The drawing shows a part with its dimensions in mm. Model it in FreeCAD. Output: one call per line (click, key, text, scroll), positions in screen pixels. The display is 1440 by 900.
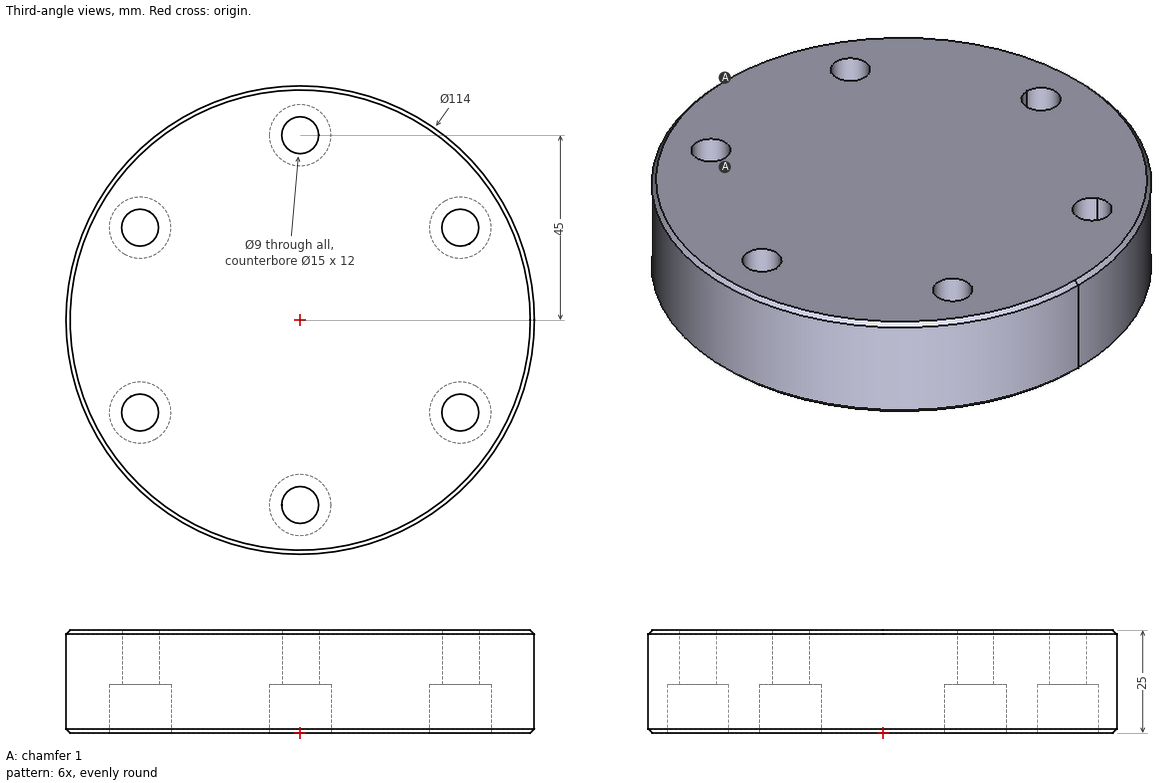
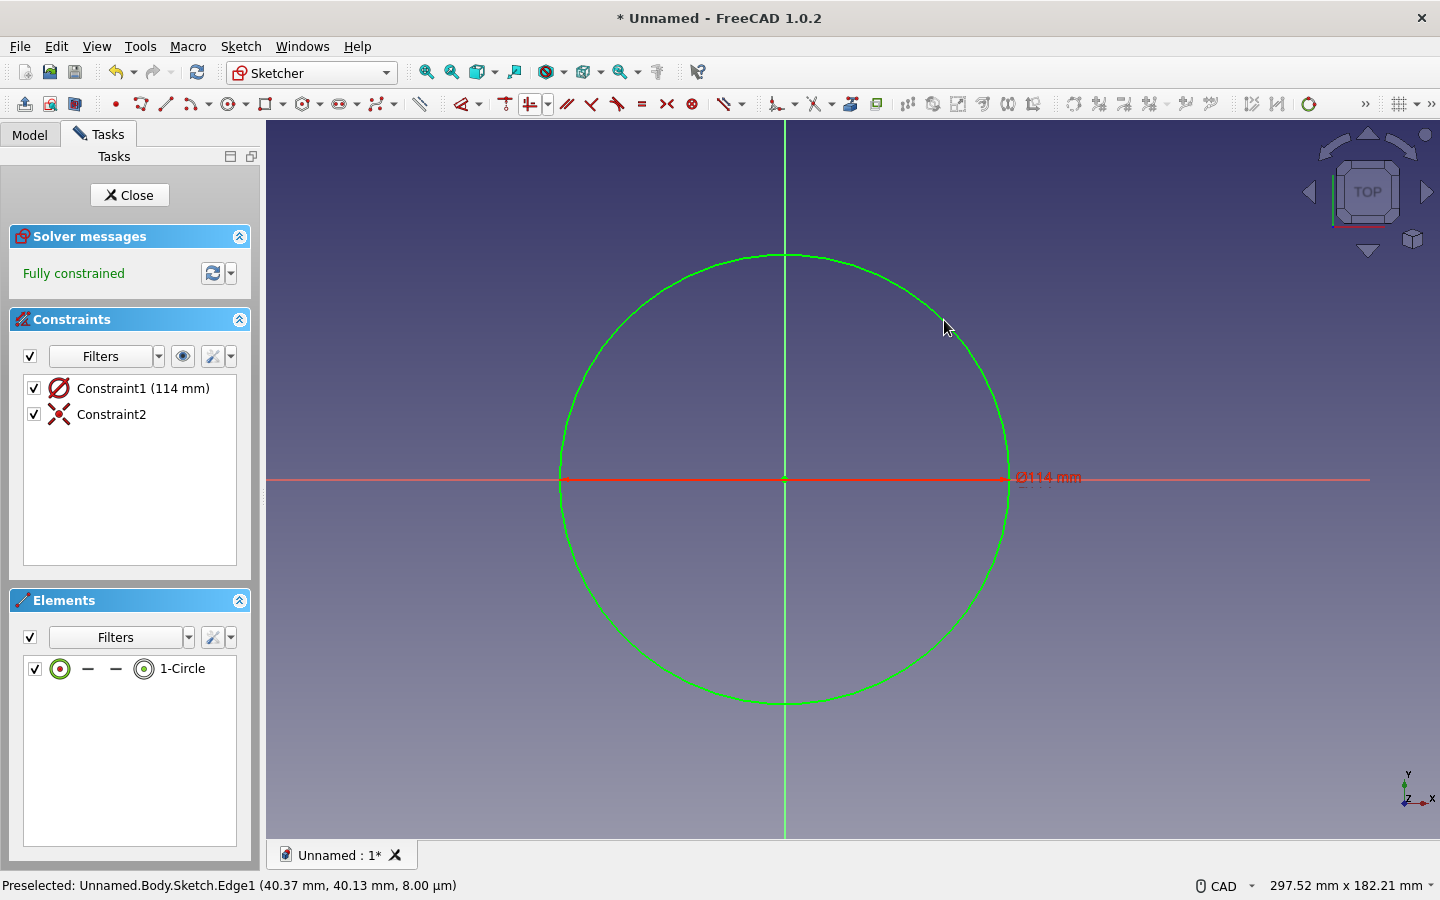
click(130, 195)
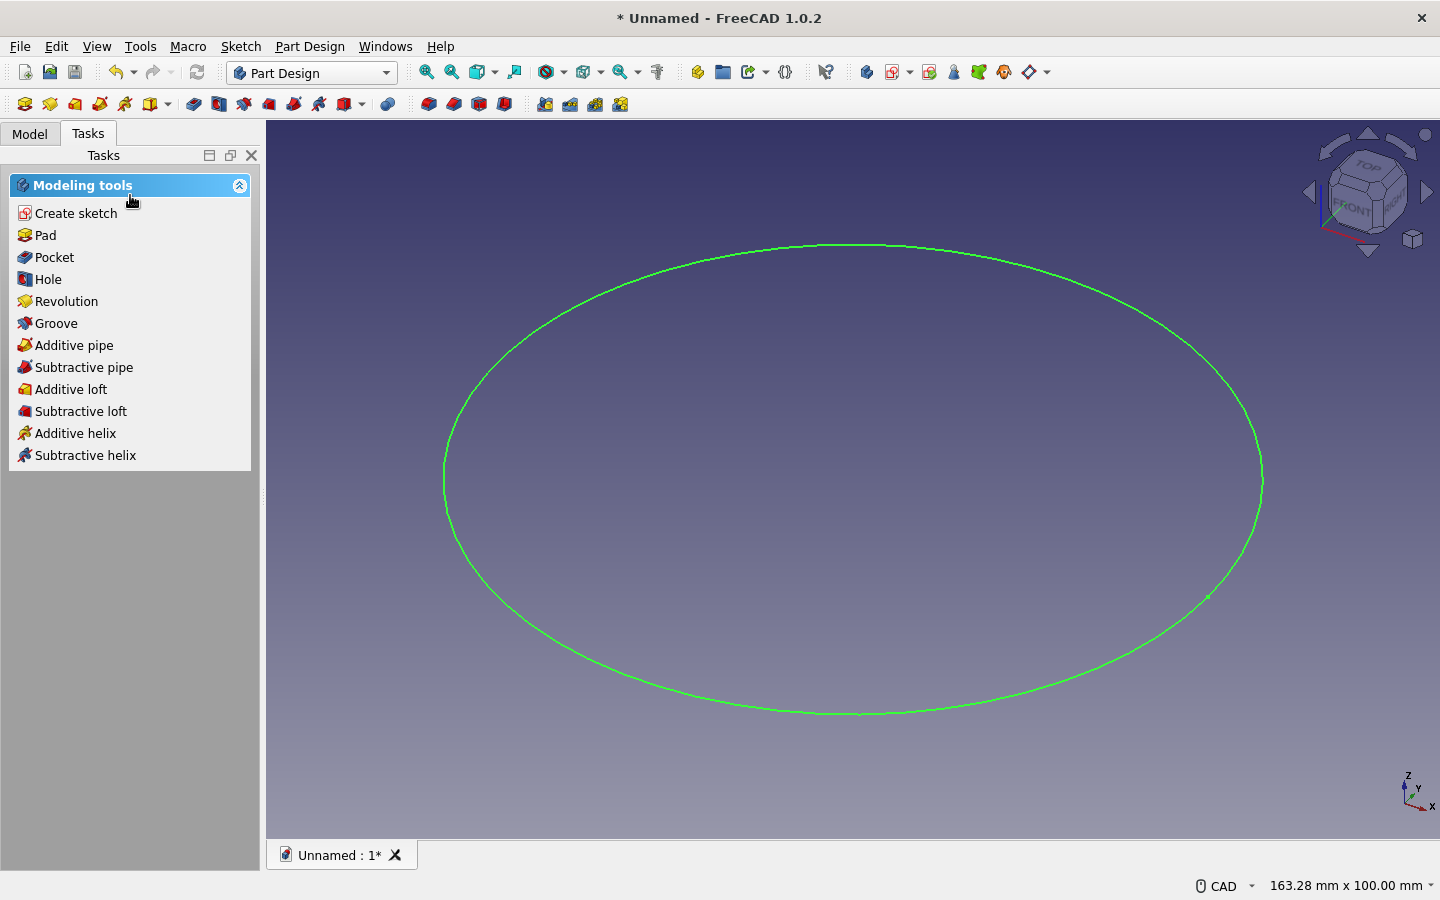
click(25, 104)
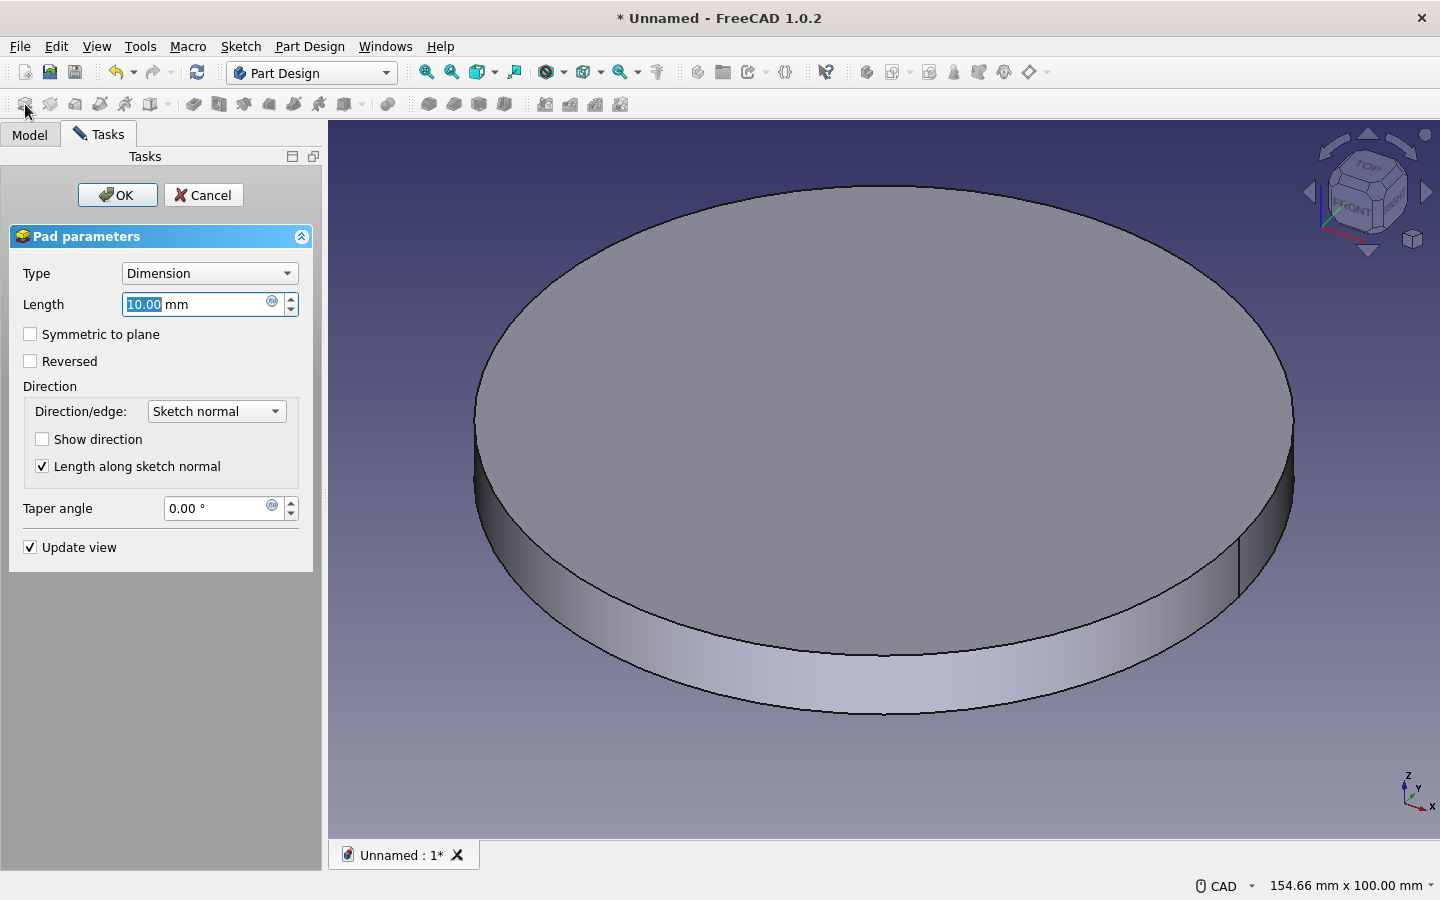
text(25)
key(Tab)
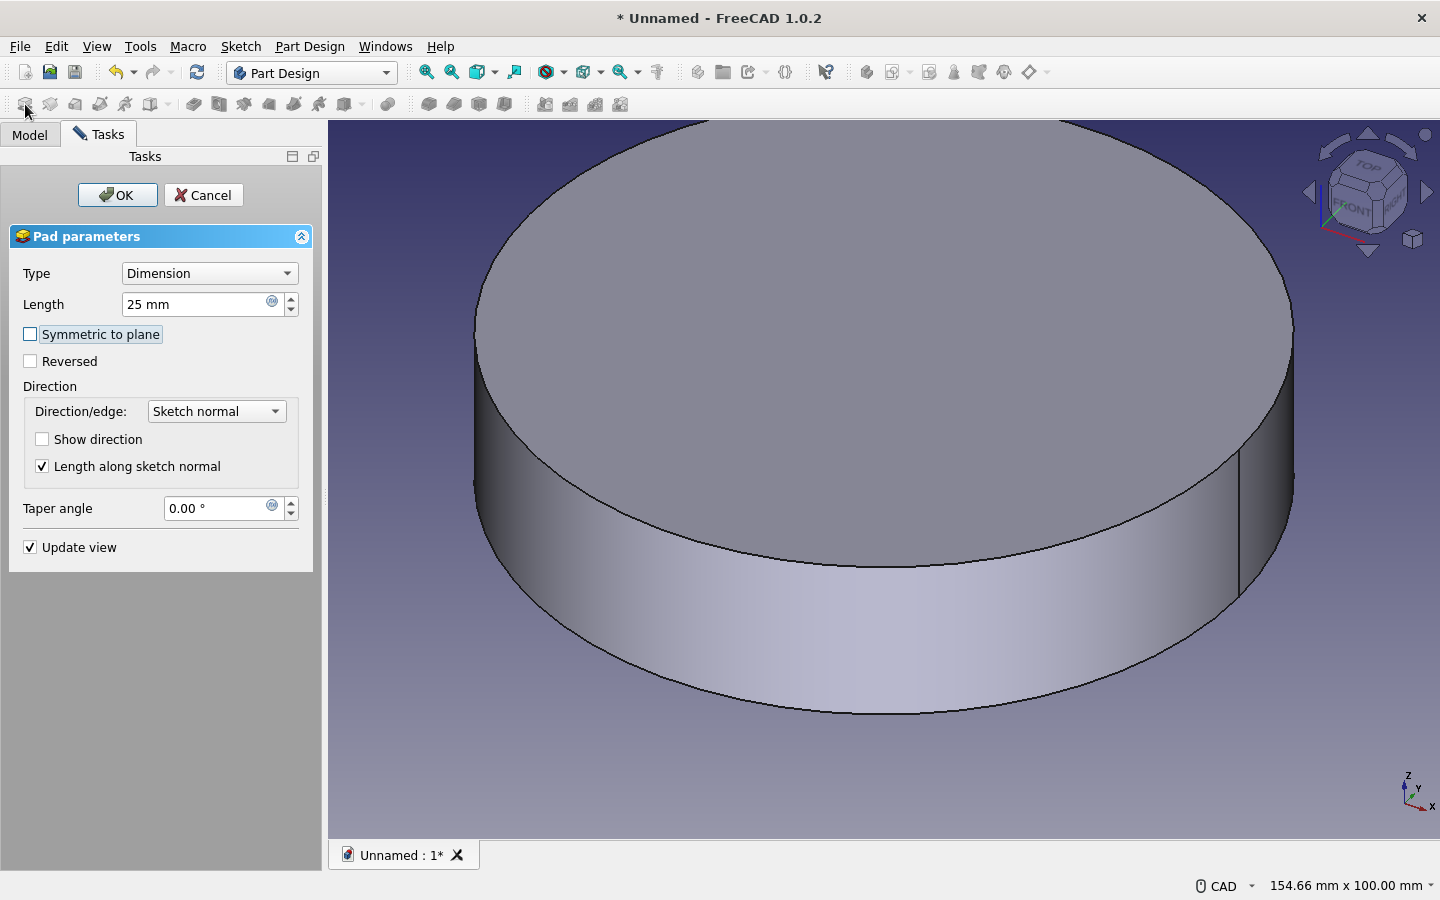
click(118, 195)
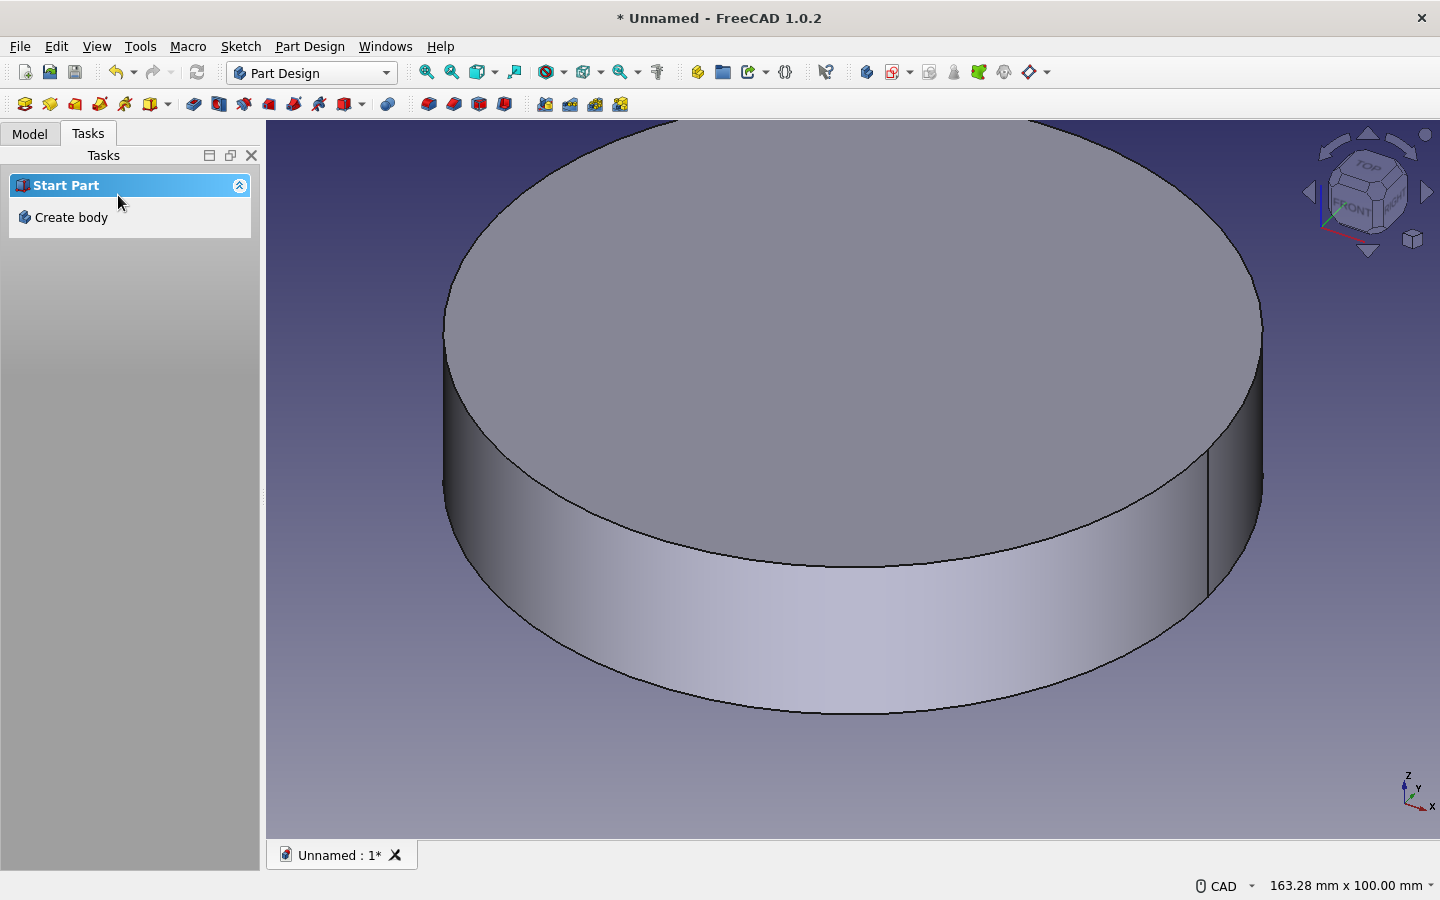
click(427, 72)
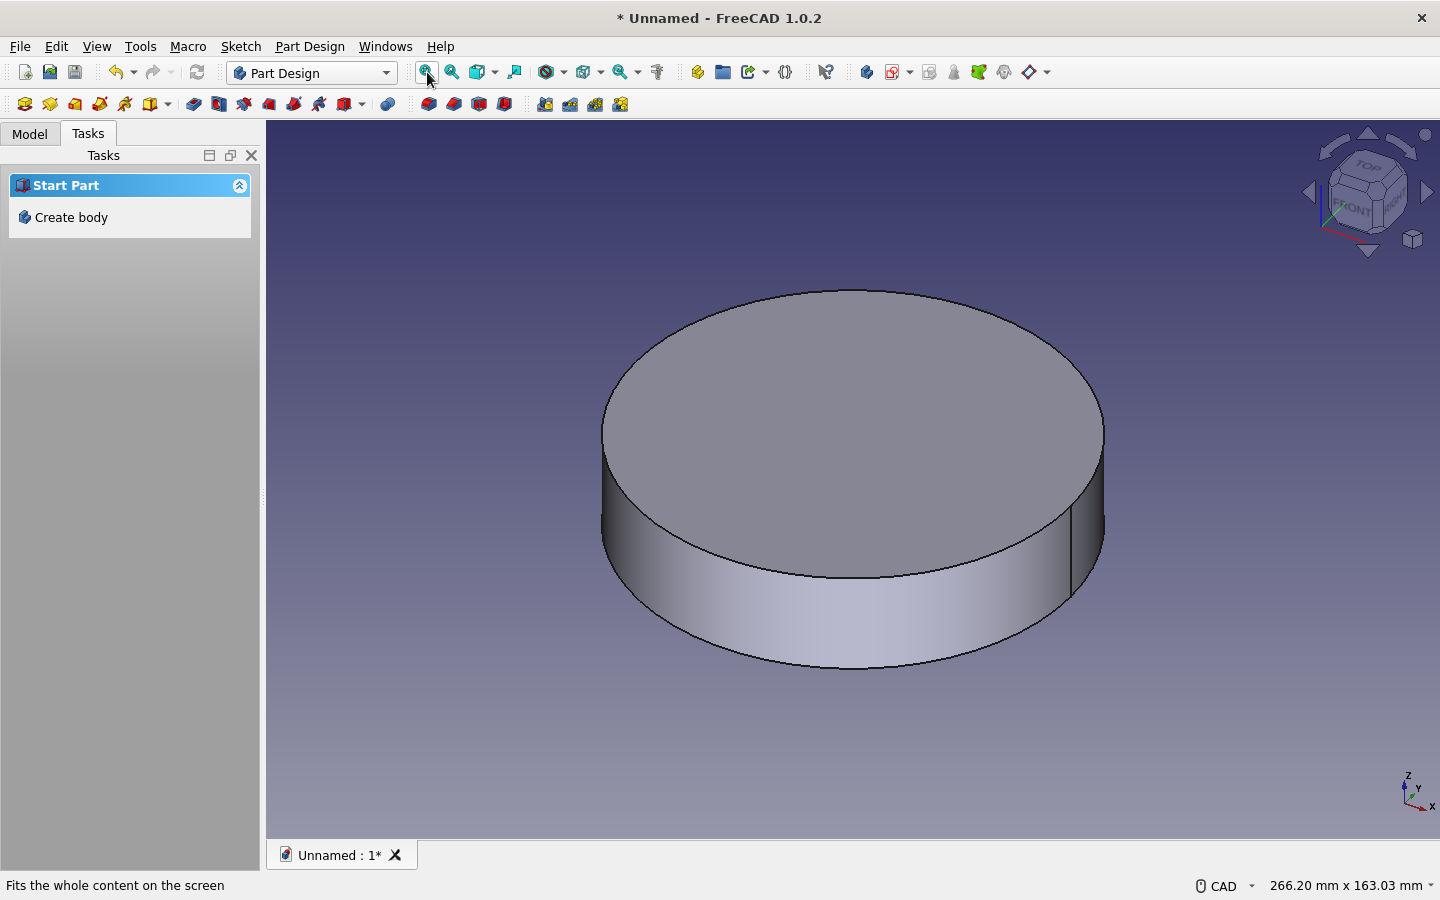
click(603, 448)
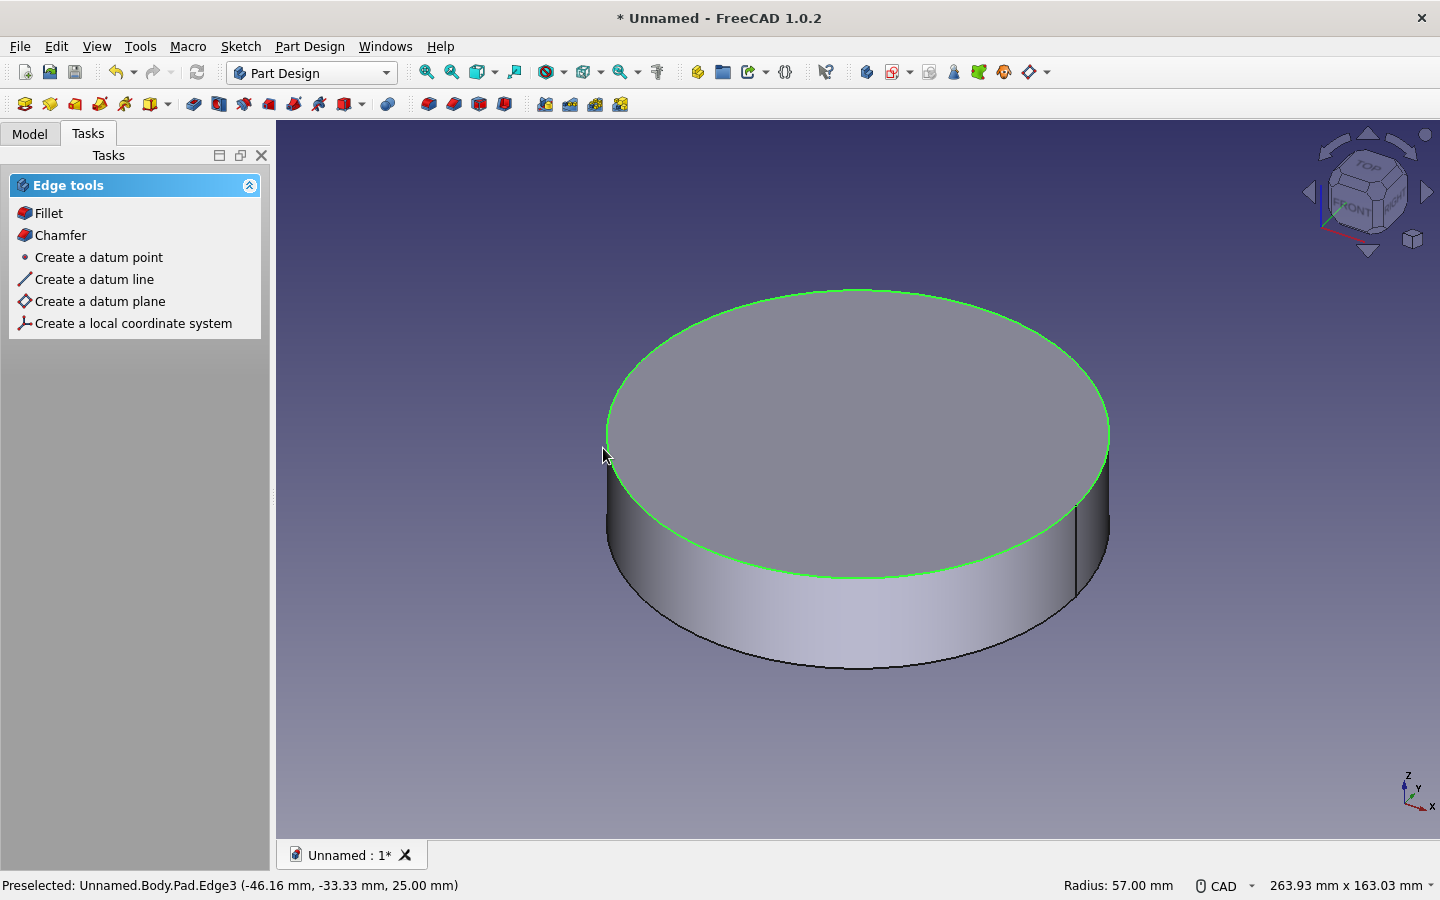
key(0)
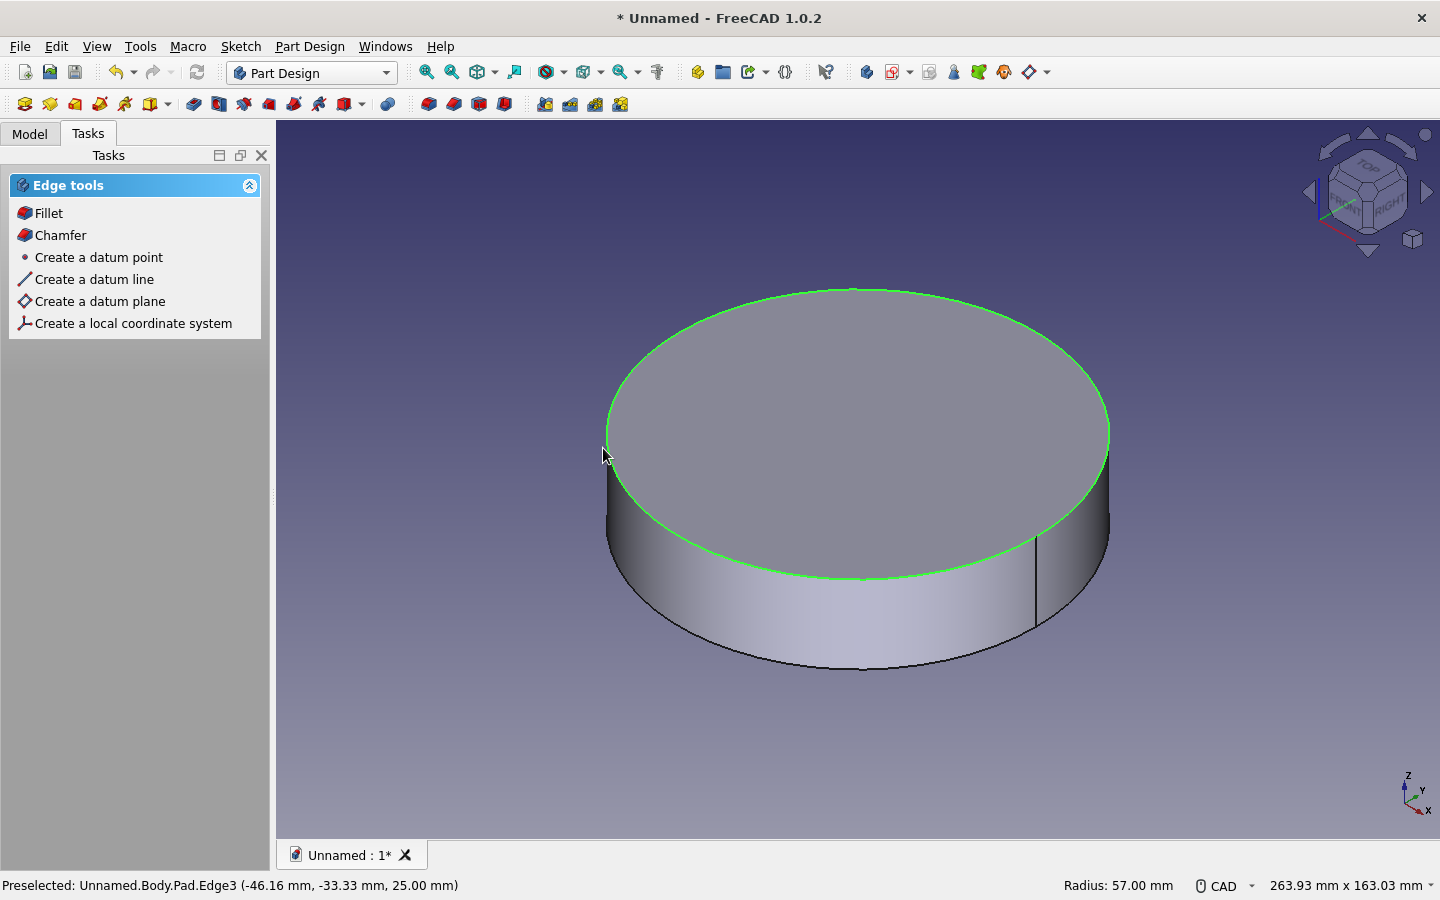
key(2)